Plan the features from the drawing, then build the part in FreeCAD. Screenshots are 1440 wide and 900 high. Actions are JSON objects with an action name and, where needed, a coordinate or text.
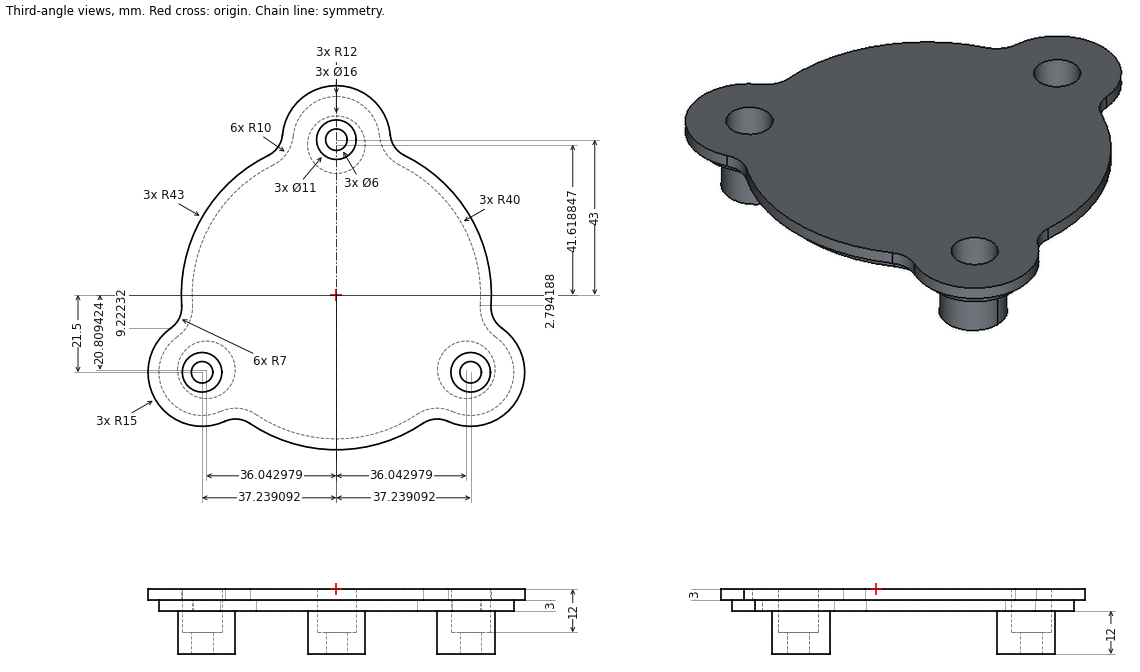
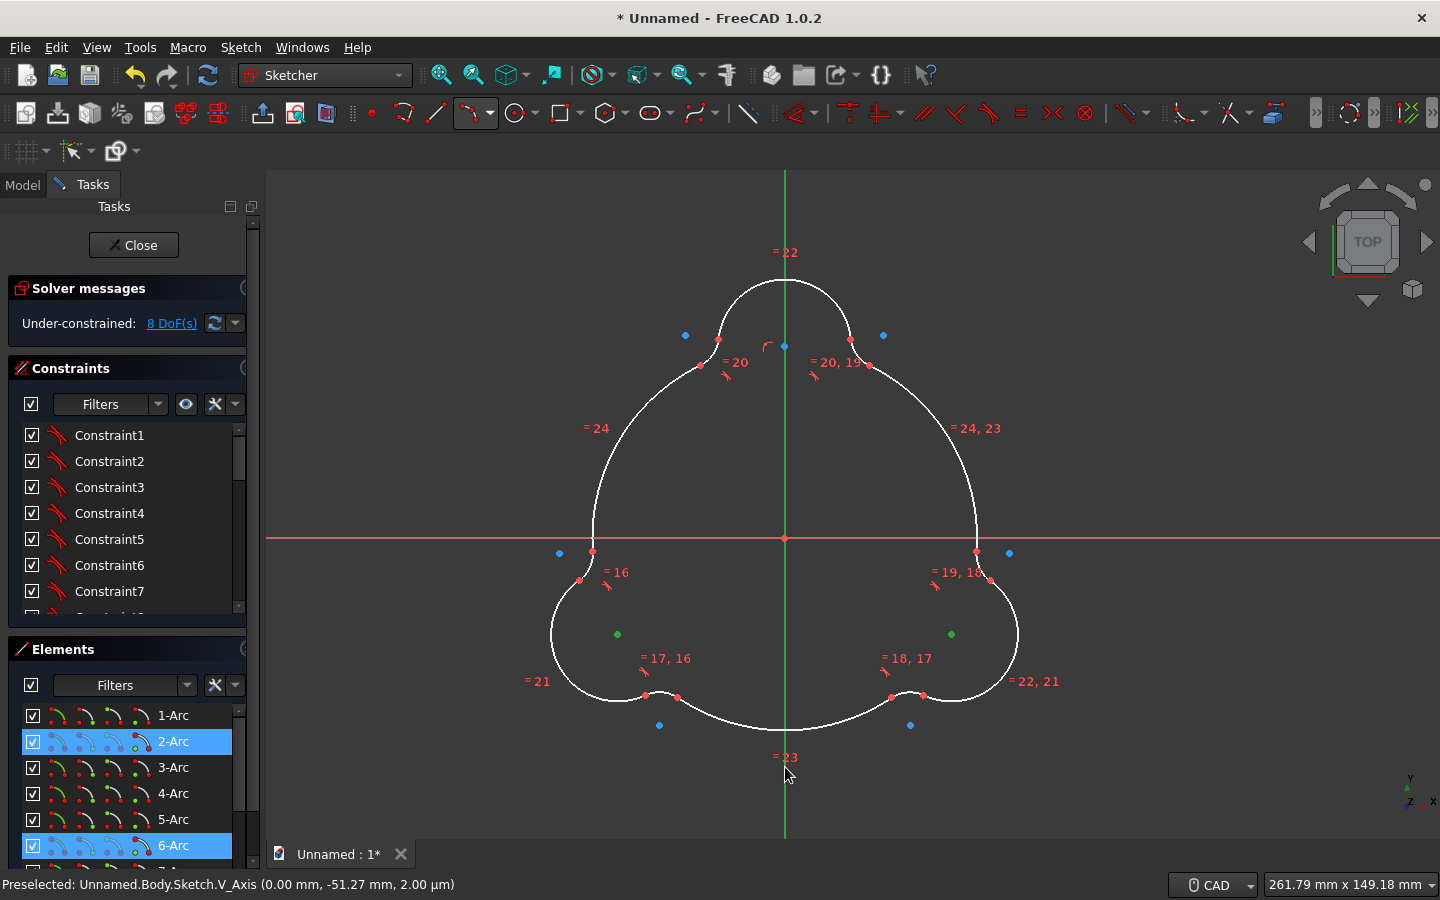
{"action": "left_click", "coordinate": [1054, 114]}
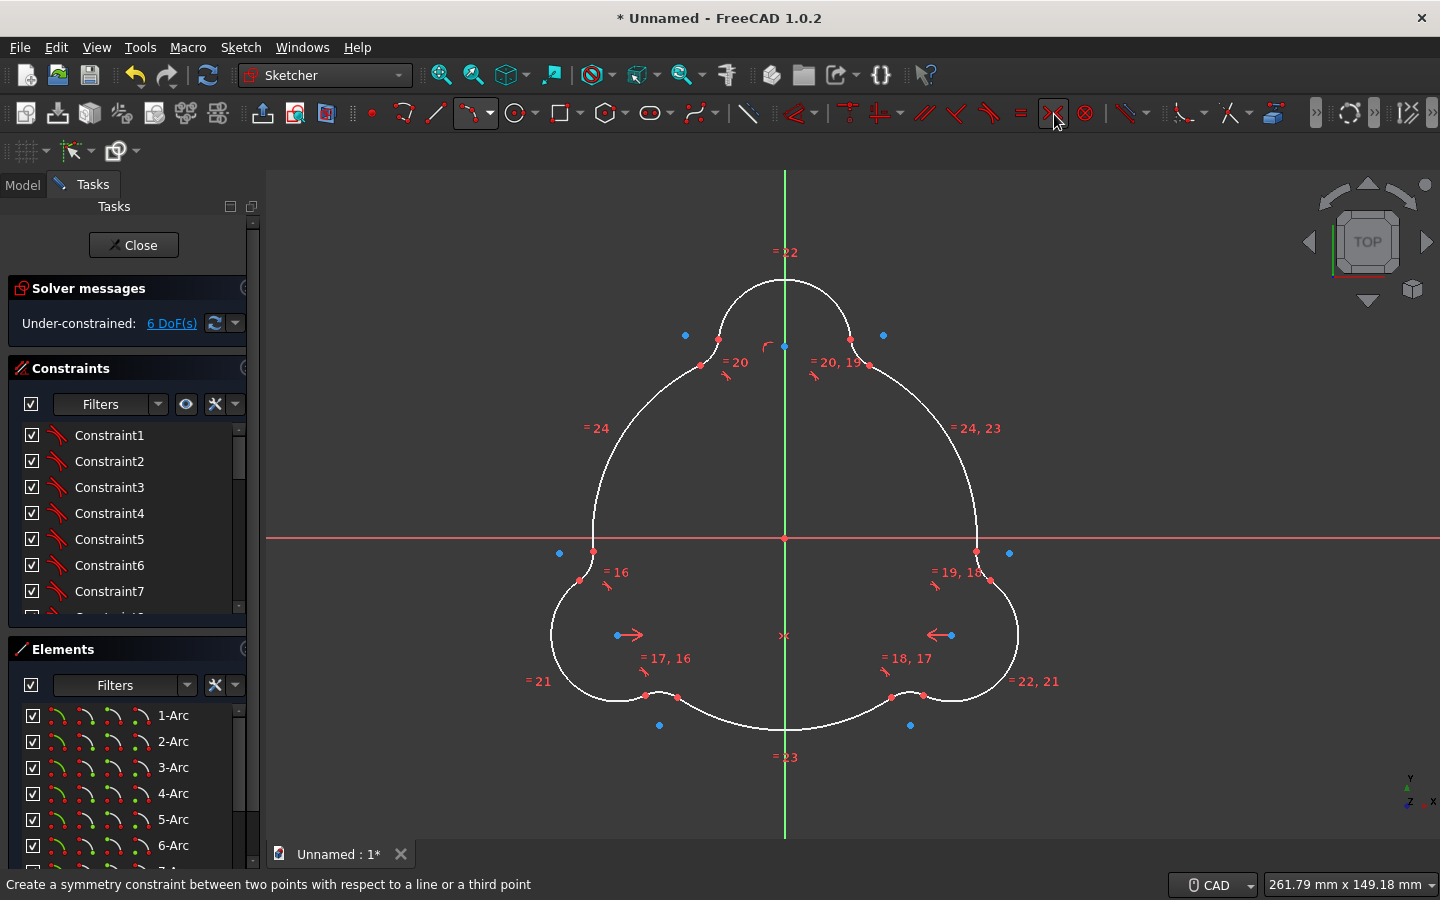
{"action": "scroll", "coordinate": [586, 574], "scroll_direction": "up", "scroll_amount": 2}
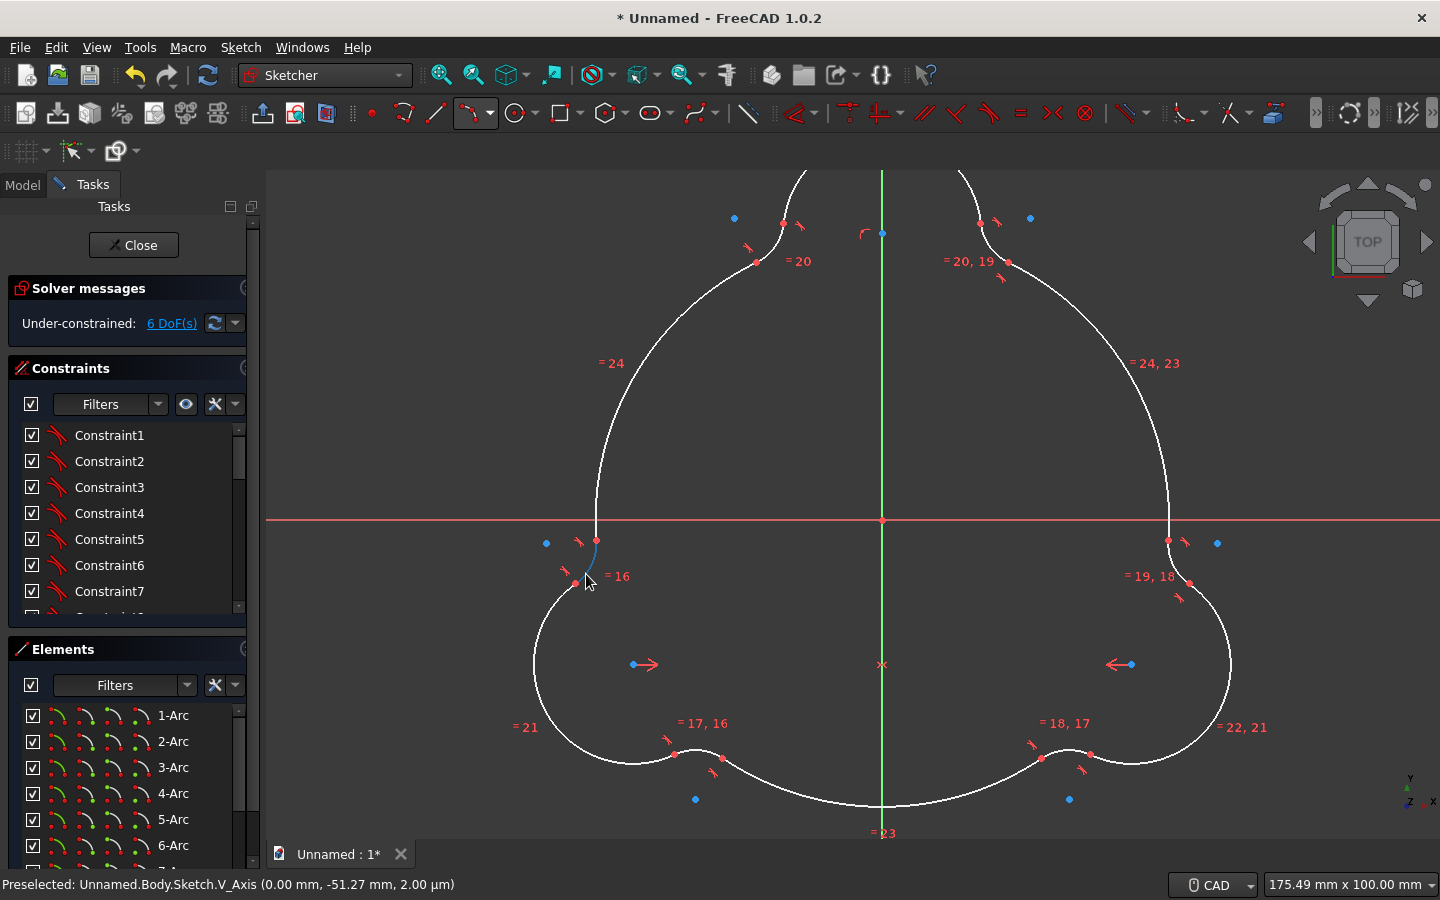
{"action": "left_click", "coordinate": [586, 573]}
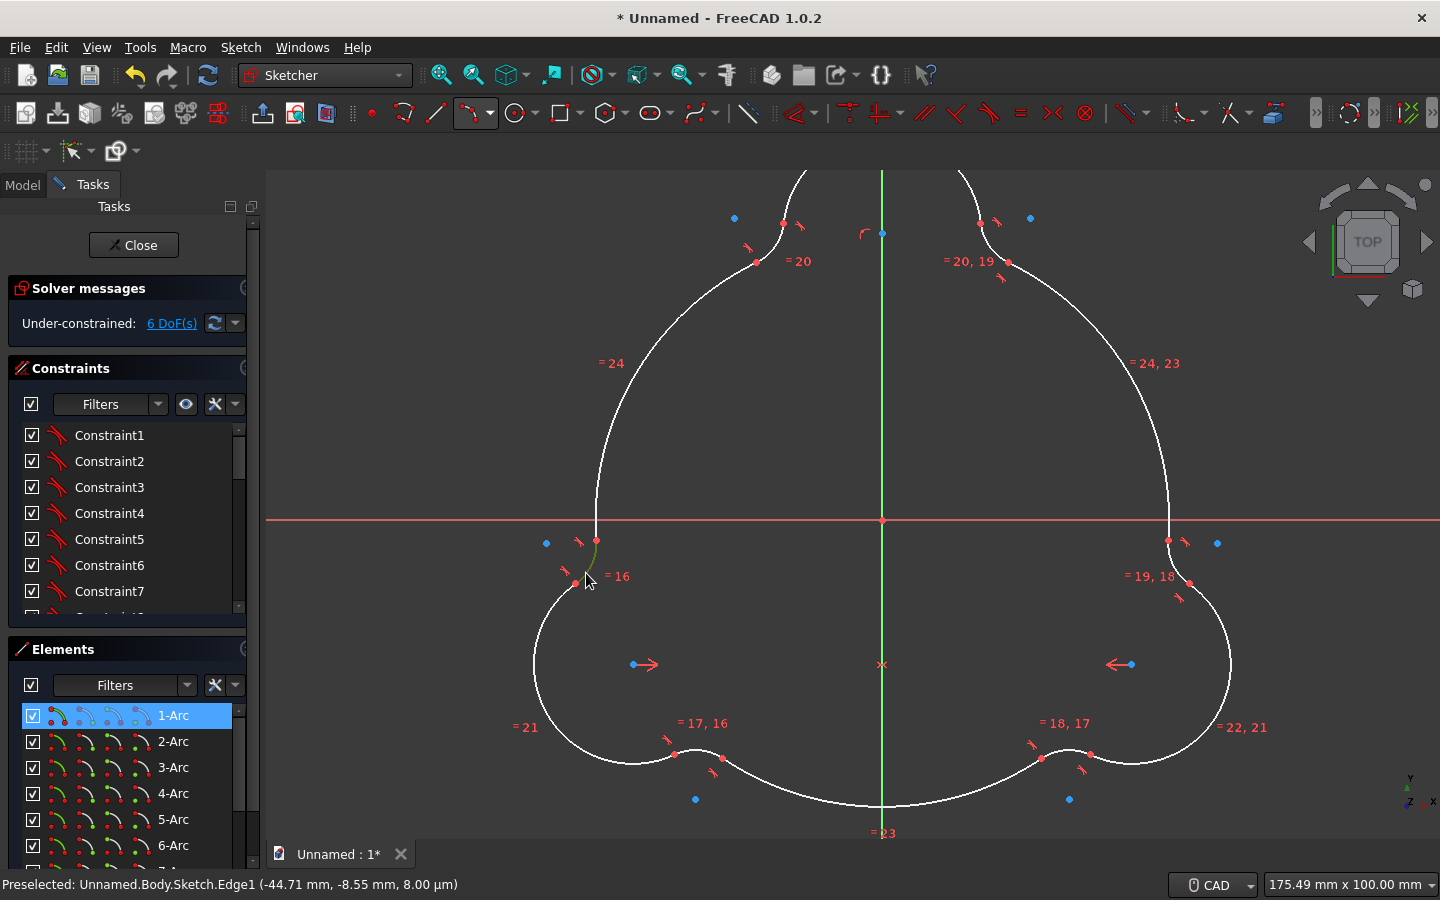
{"action": "left_click", "coordinate": [816, 114]}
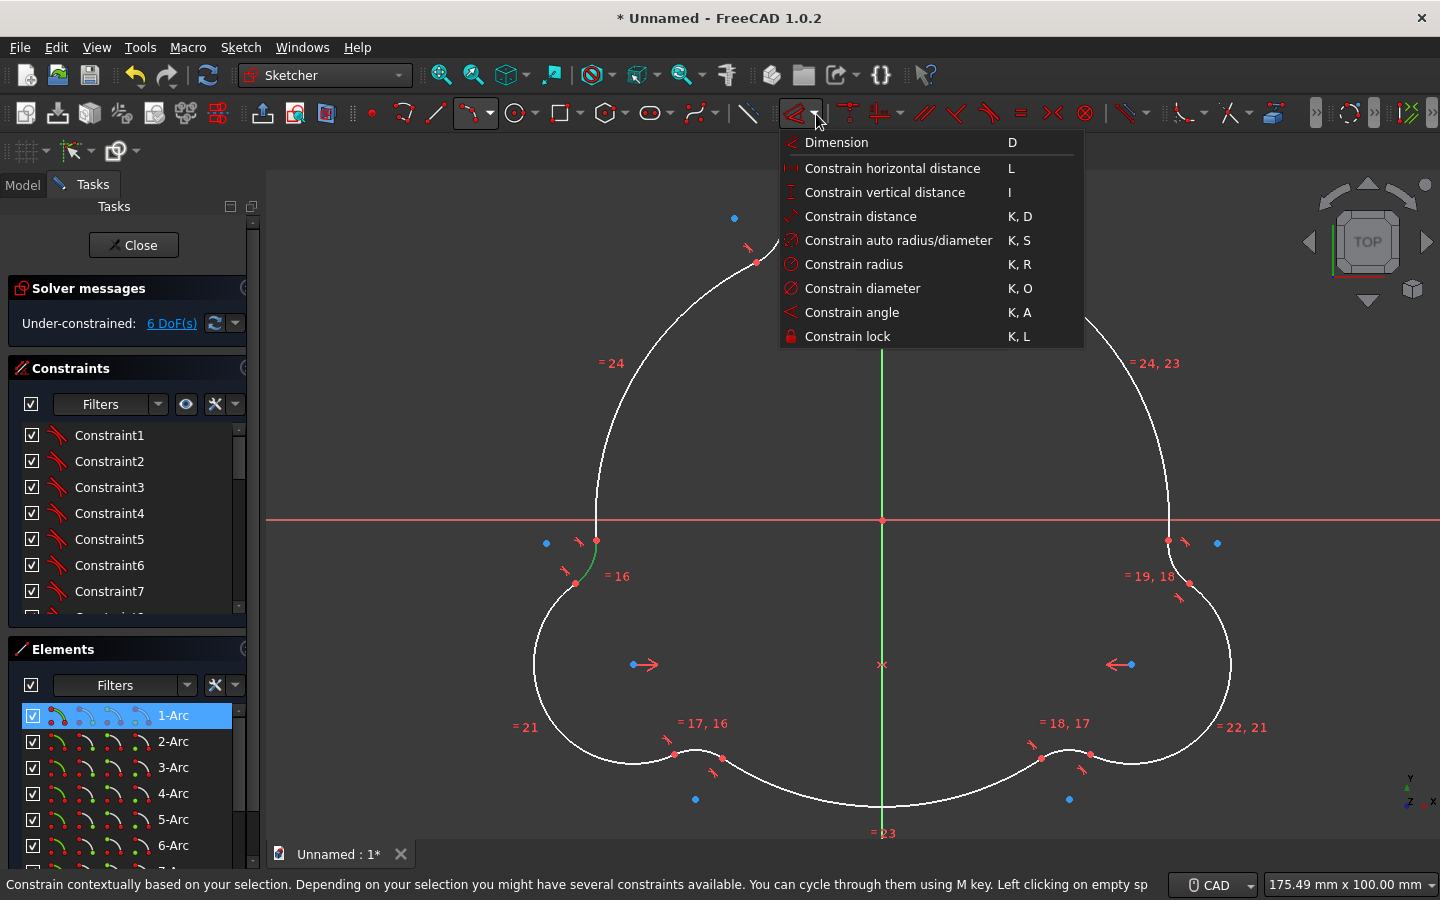
{"action": "left_click", "coordinate": [932, 264]}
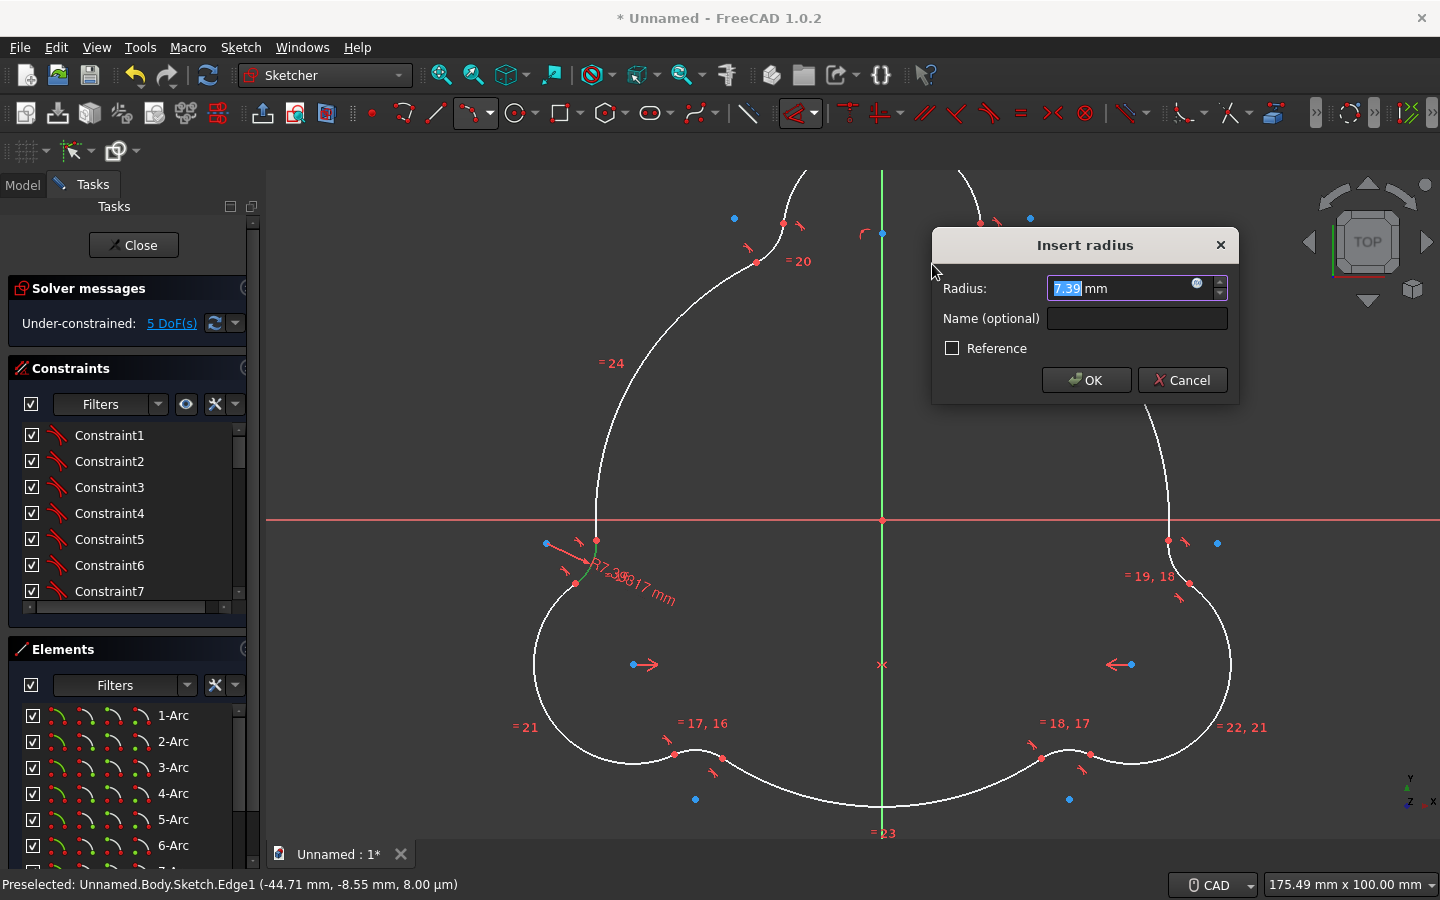
{"action": "type", "text": "7"}
{"action": "key", "text": "Return"}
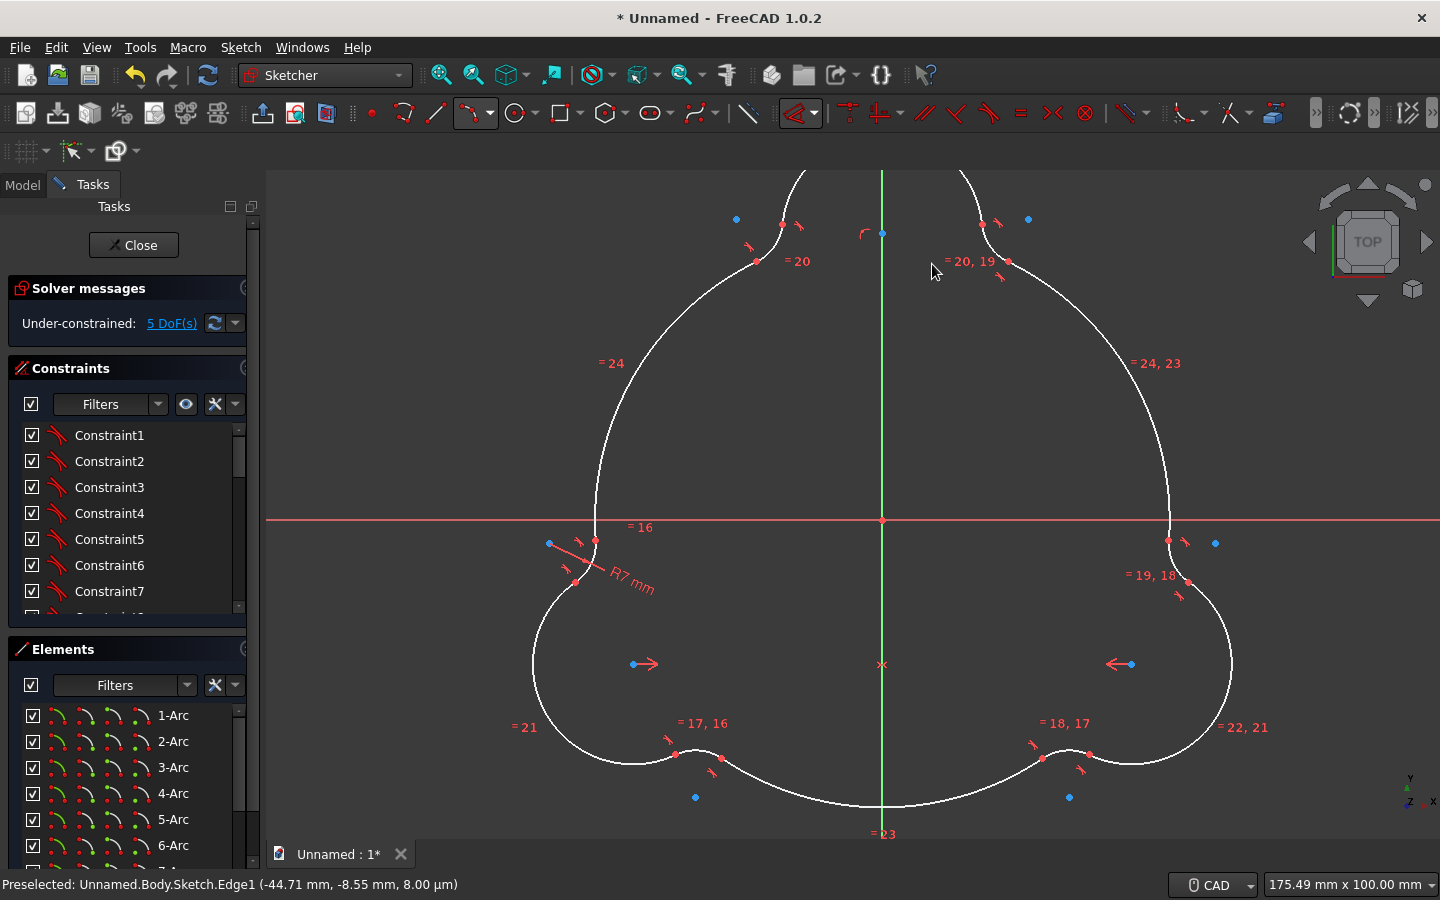
{"action": "left_click", "coordinate": [533, 657]}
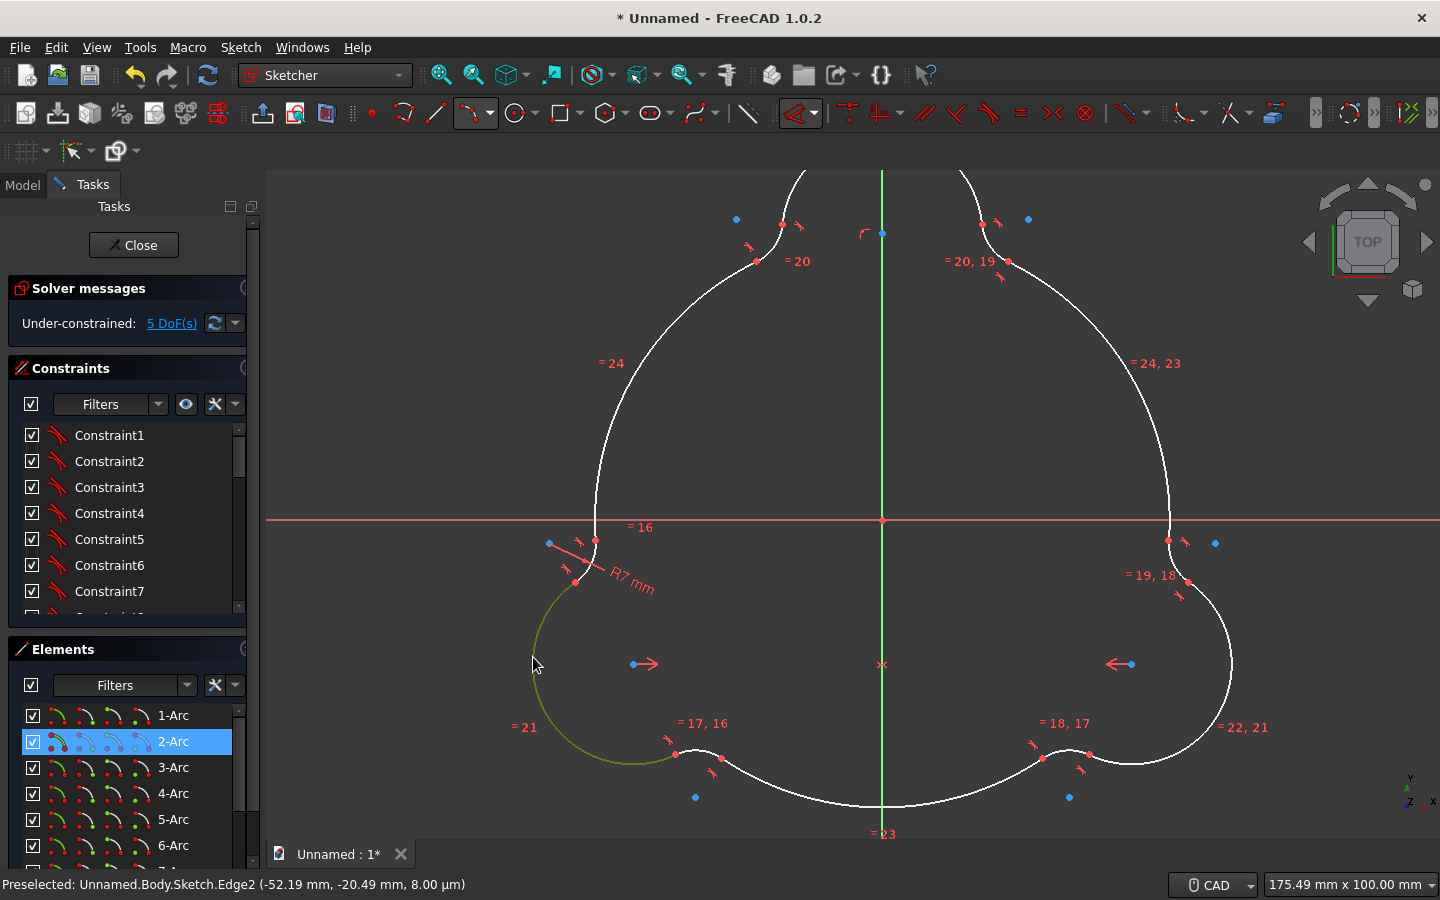
{"action": "left_click", "coordinate": [816, 114]}